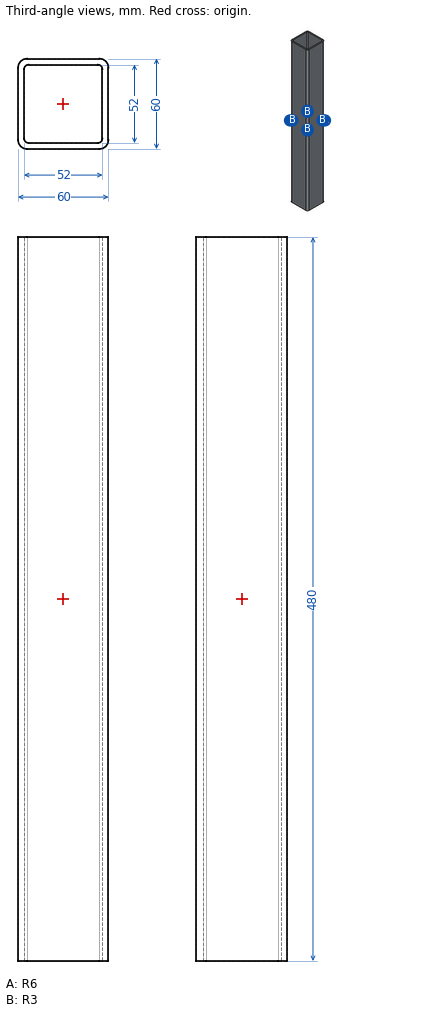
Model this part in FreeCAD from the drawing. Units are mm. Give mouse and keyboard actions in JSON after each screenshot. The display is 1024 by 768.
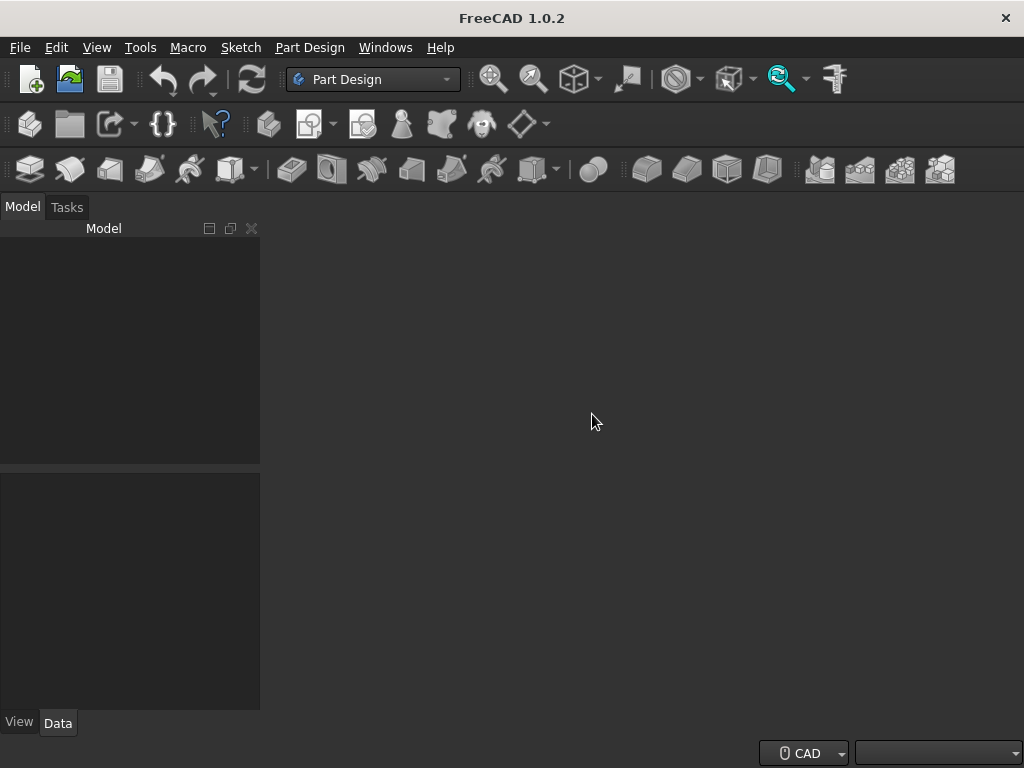
{"action": "left_click", "coordinate": [30, 80]}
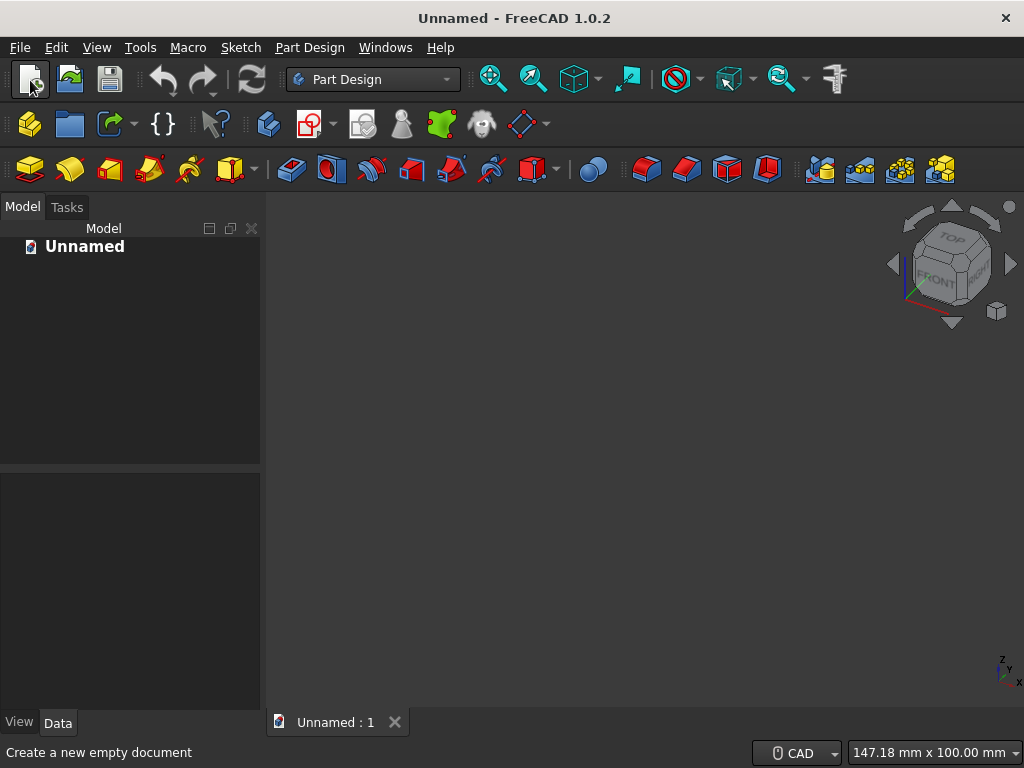
{"action": "left_click", "coordinate": [310, 124]}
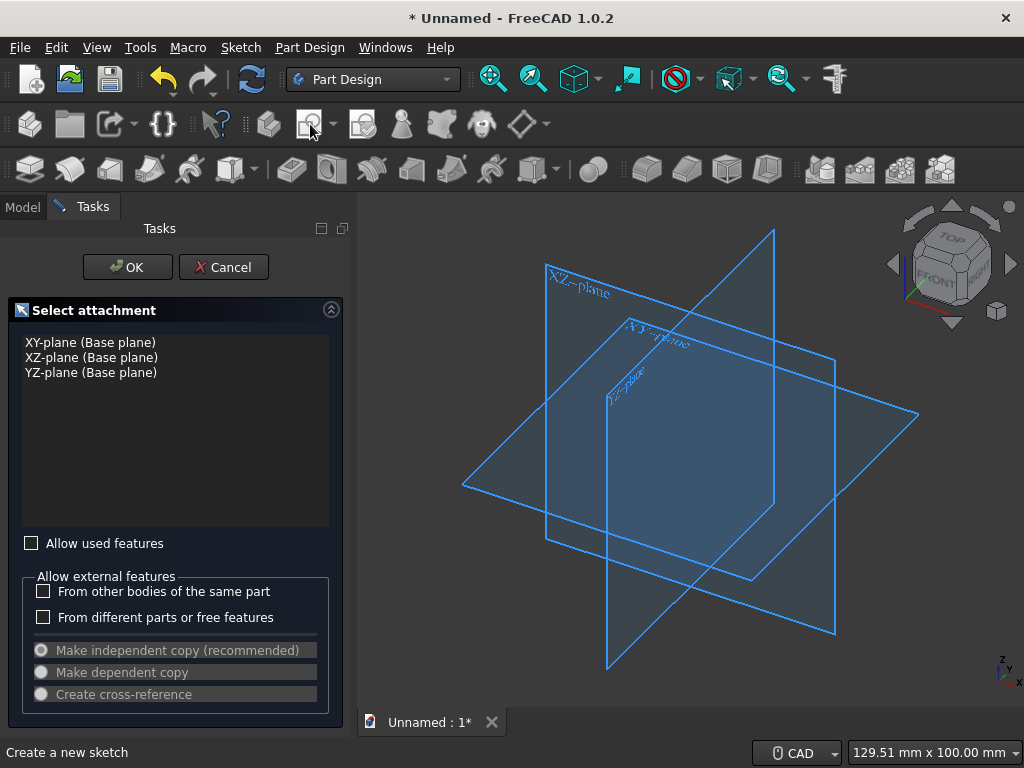
{"action": "left_click", "coordinate": [82, 342]}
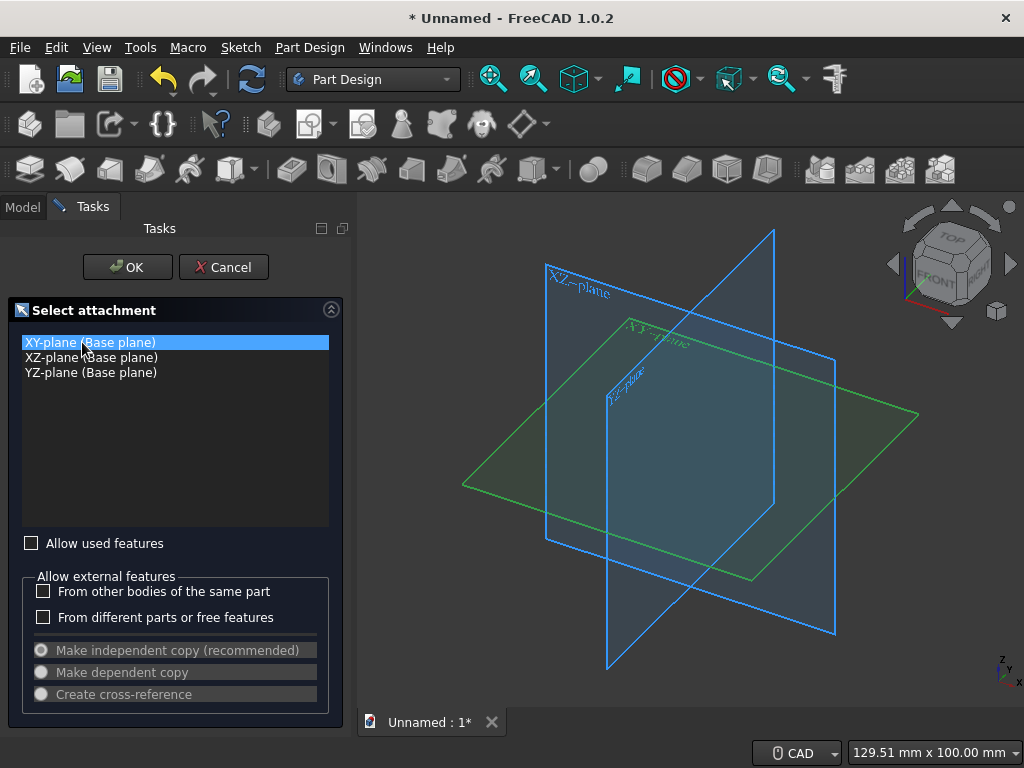
{"action": "left_click", "coordinate": [128, 267]}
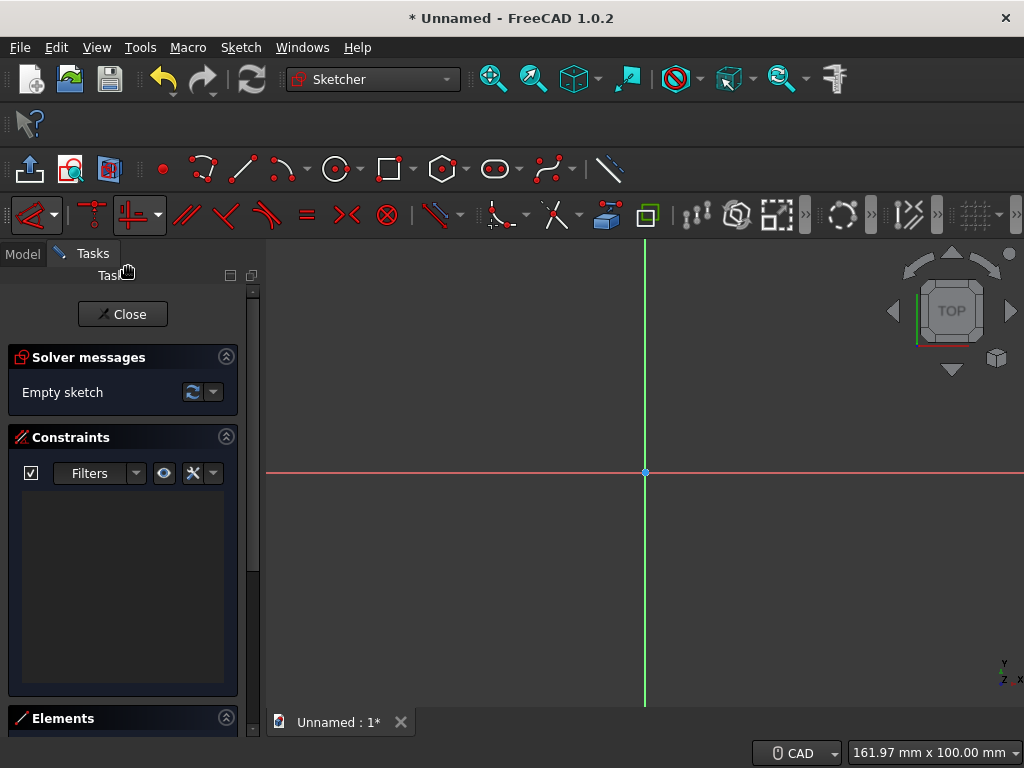
{"action": "key", "text": "g v"}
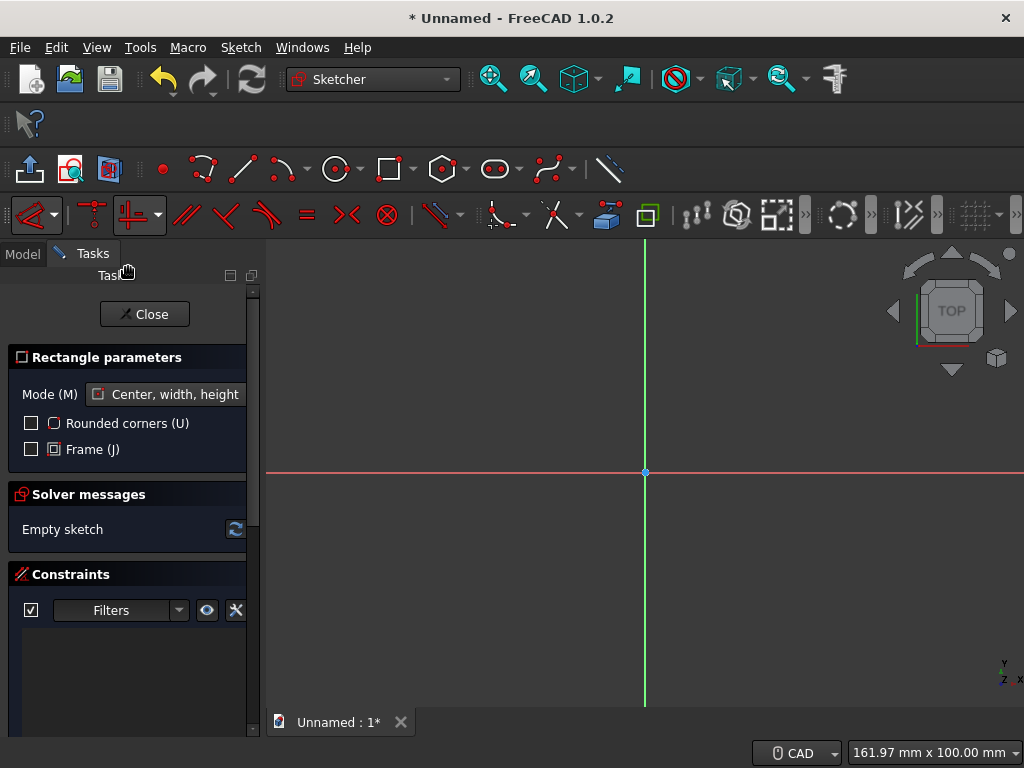
{"action": "left_click", "coordinate": [645, 473]}
{"action": "mouse_move", "coordinate": [785, 333]}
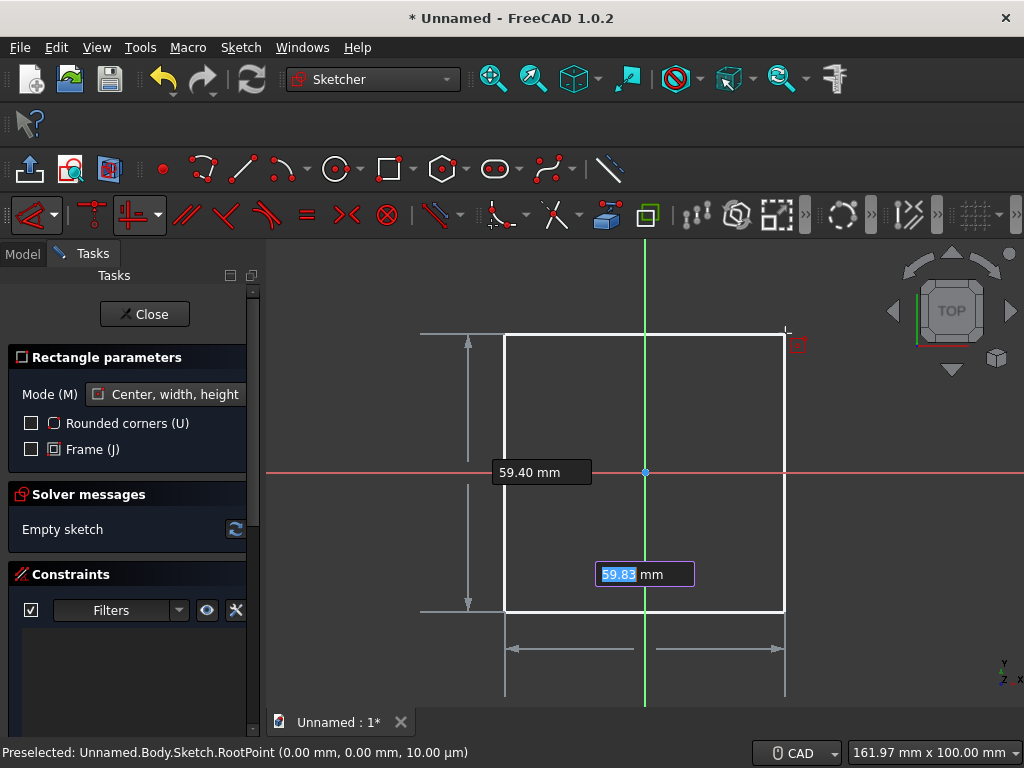
{"action": "type", "text": "60"}
{"action": "key", "text": "Tab"}
{"action": "type", "text": "60"}
{"action": "key", "text": "Return"}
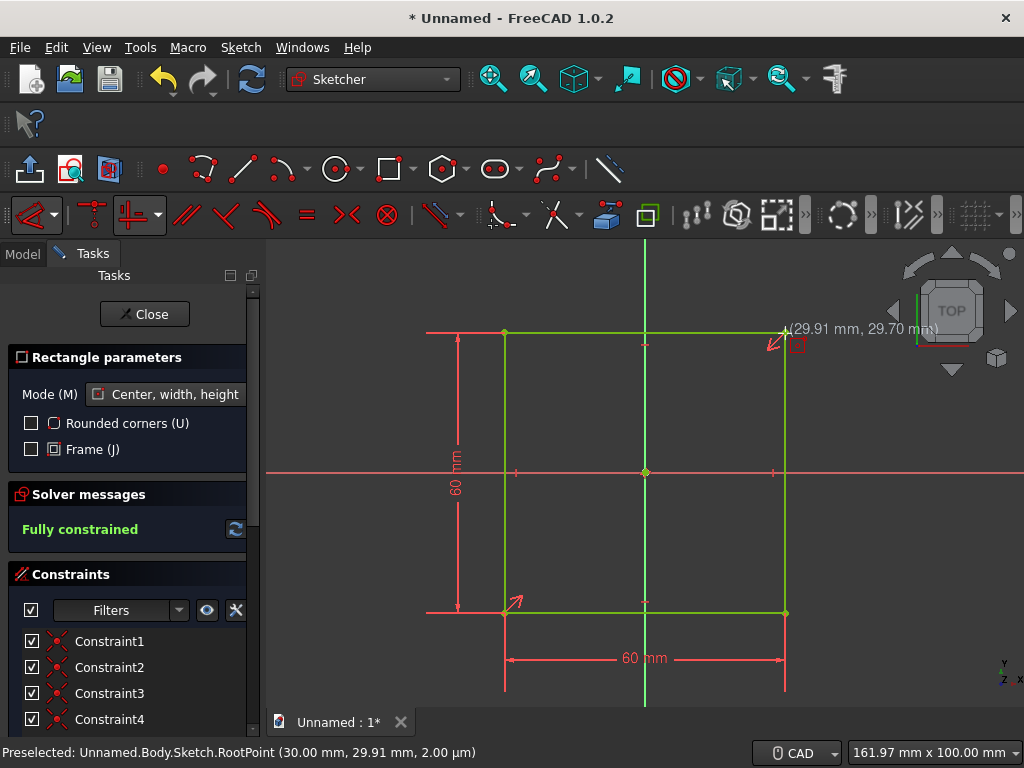
{"action": "left_click", "coordinate": [645, 473]}
{"action": "mouse_move", "coordinate": [767, 351]}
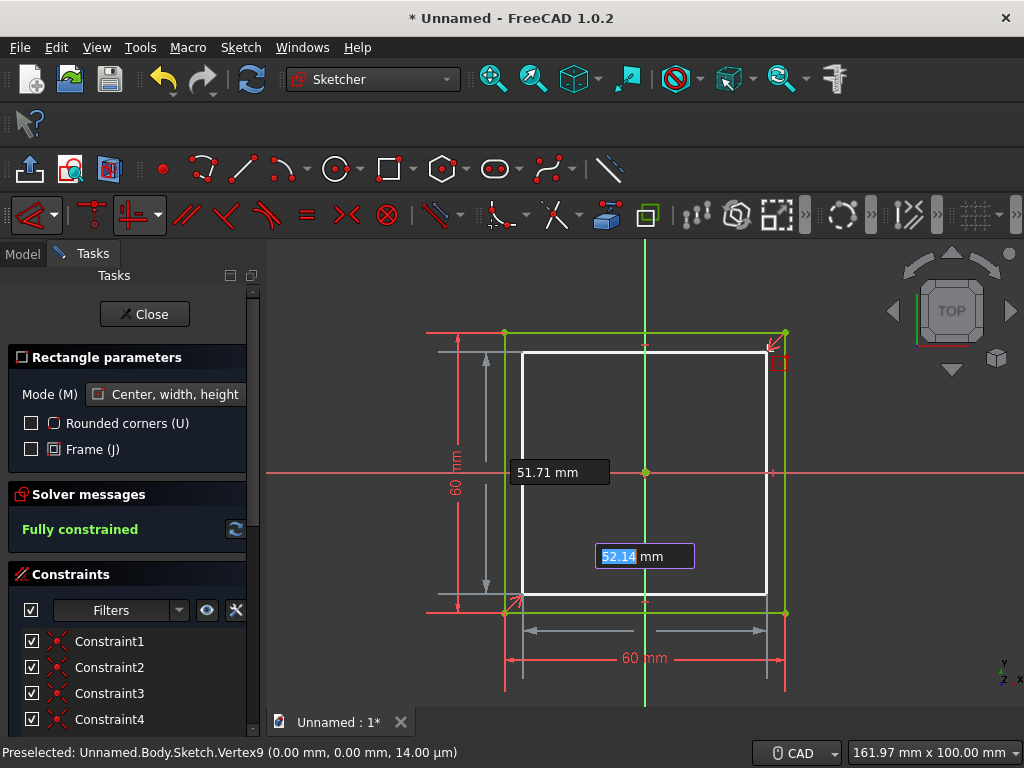
{"action": "type", "text": "52"}
{"action": "key", "text": "Tab"}
{"action": "type", "text": "52"}
{"action": "key", "text": "Return"}
{"action": "key", "text": "Escape"}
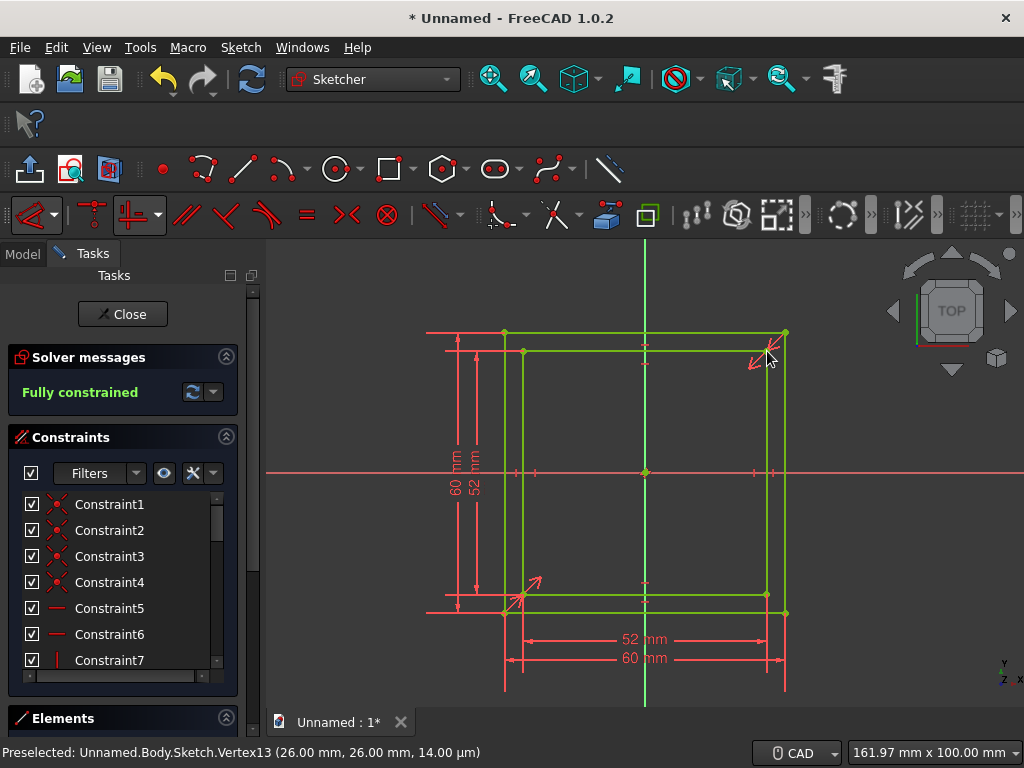
{"action": "left_click", "coordinate": [123, 314]}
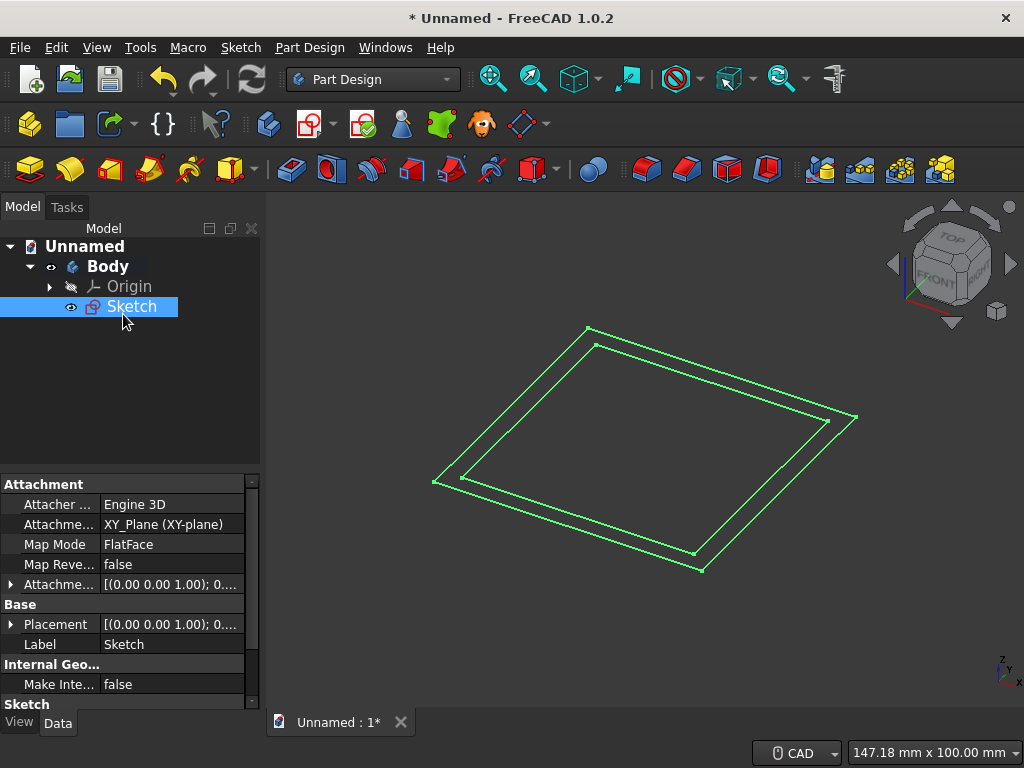
{"action": "left_click", "coordinate": [30, 170]}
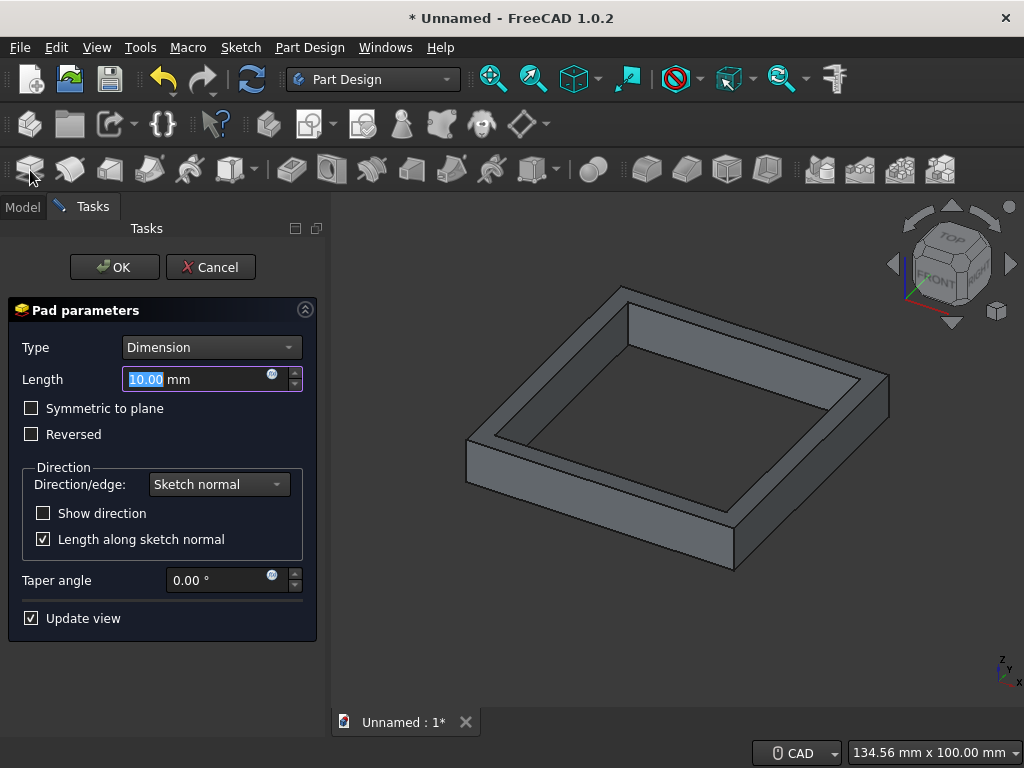
{"action": "type", "text": "480"}
{"action": "key", "text": "Tab"}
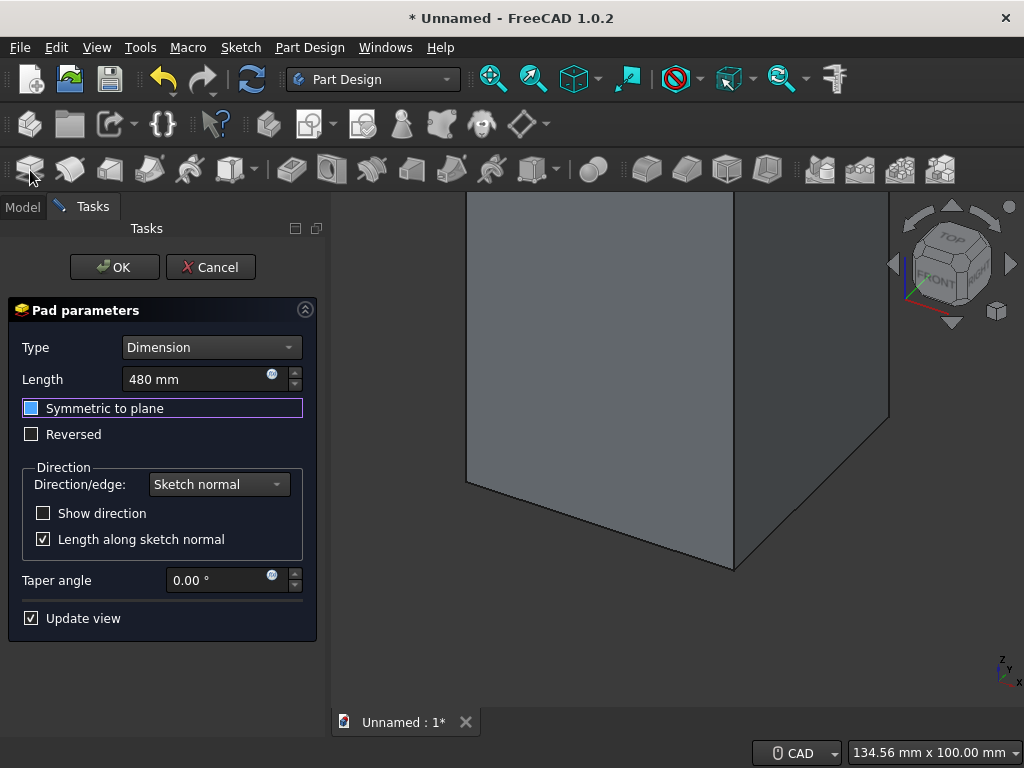
{"action": "left_click", "coordinate": [30, 408]}